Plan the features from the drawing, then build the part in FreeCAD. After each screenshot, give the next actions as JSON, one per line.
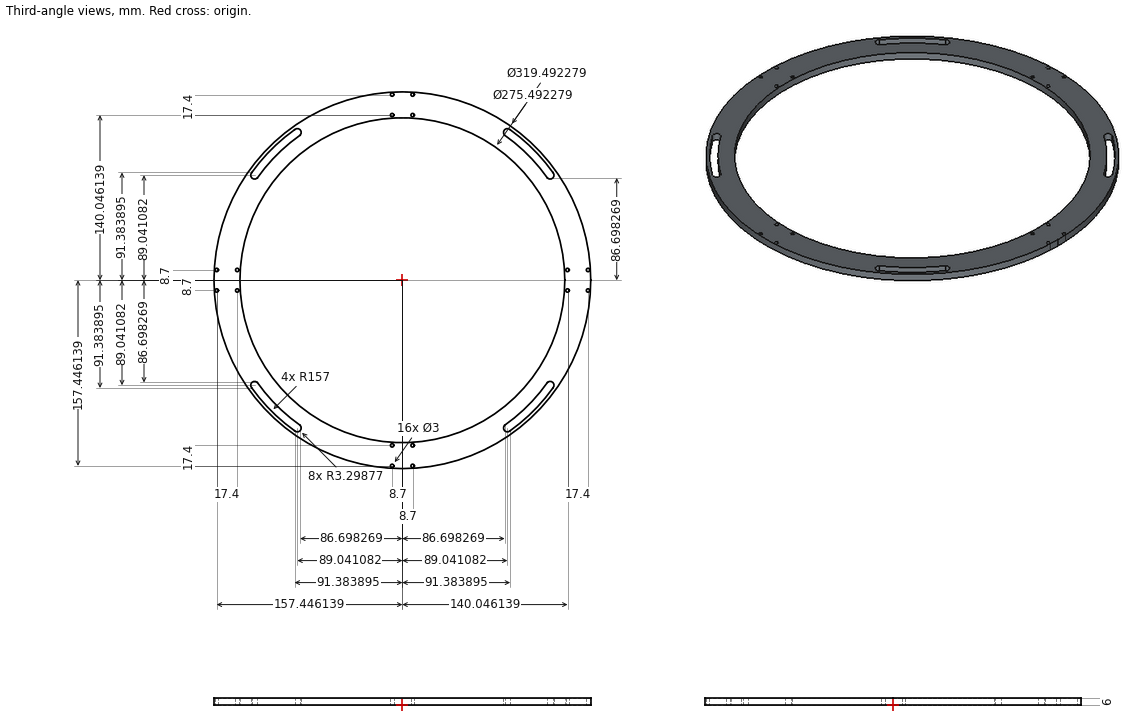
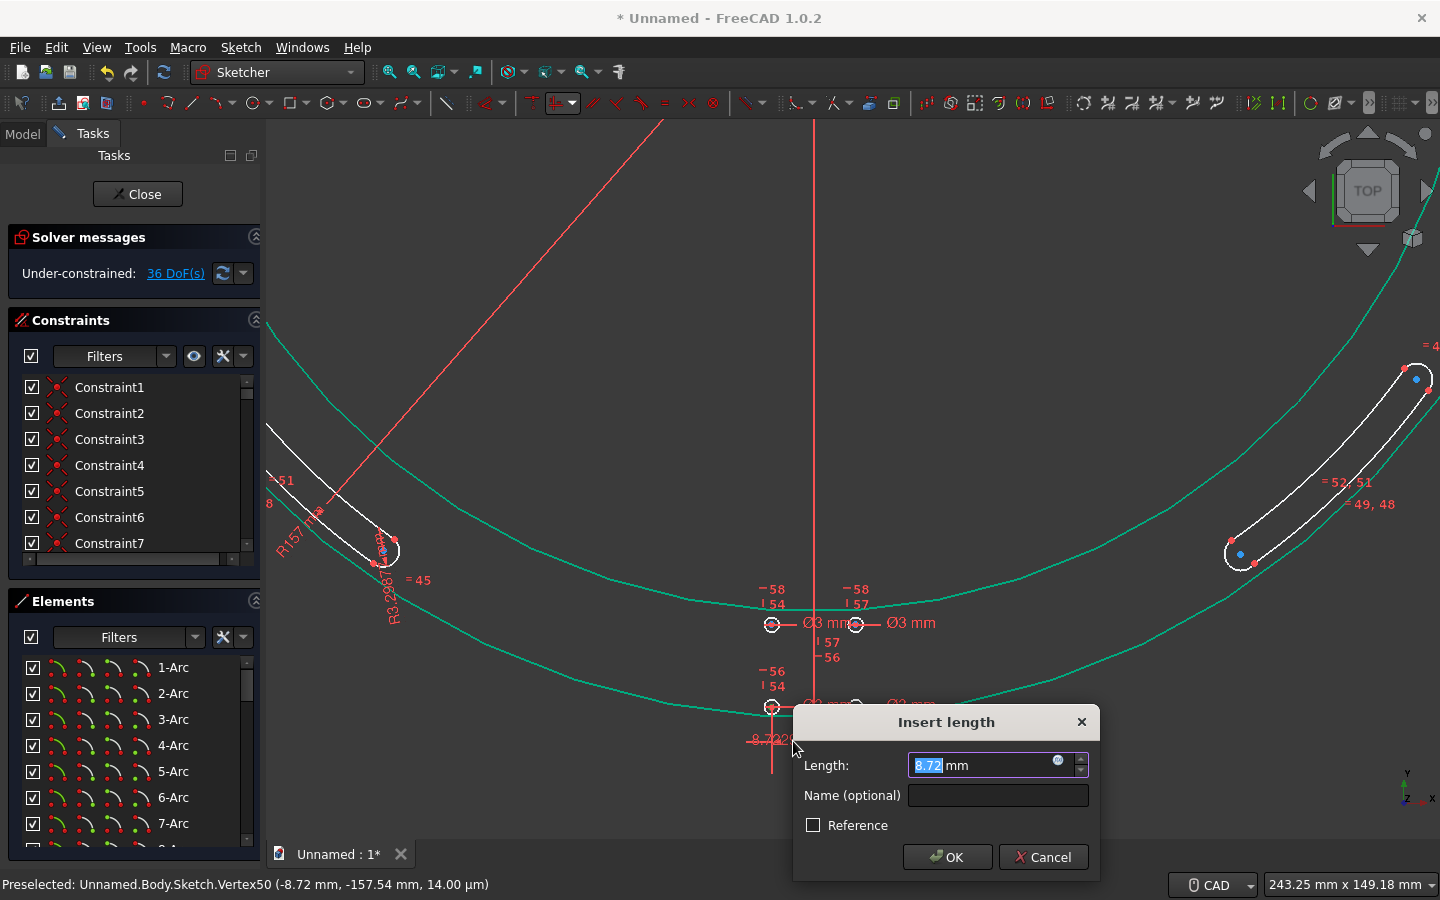
{"action": "type", "text": "8.7"}
{"action": "key", "text": "Return"}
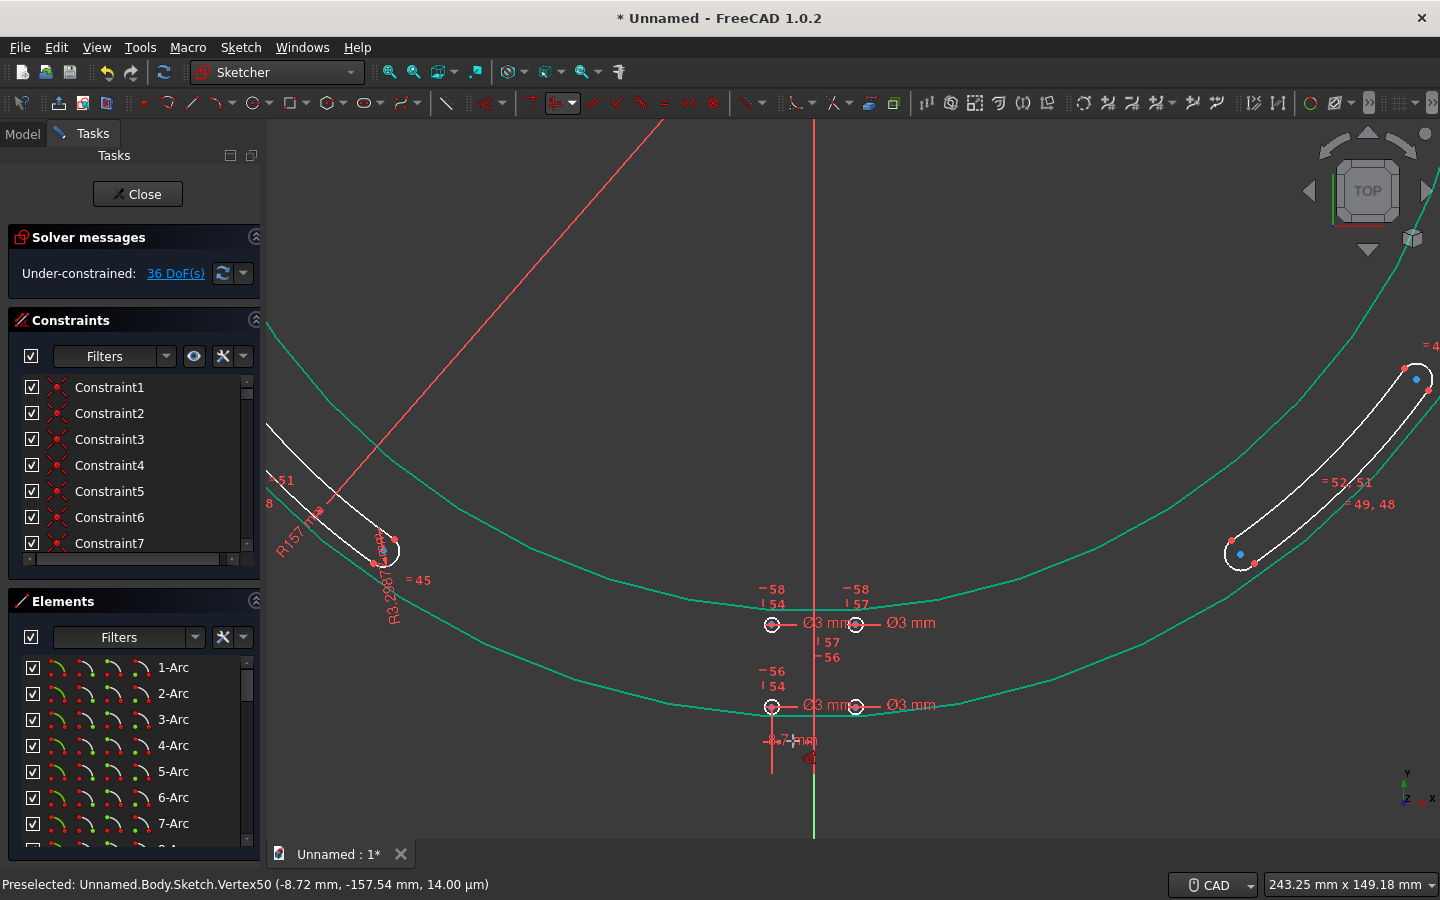
{"action": "scroll", "coordinate": [772, 708], "scroll_direction": "down", "scroll_amount": 6}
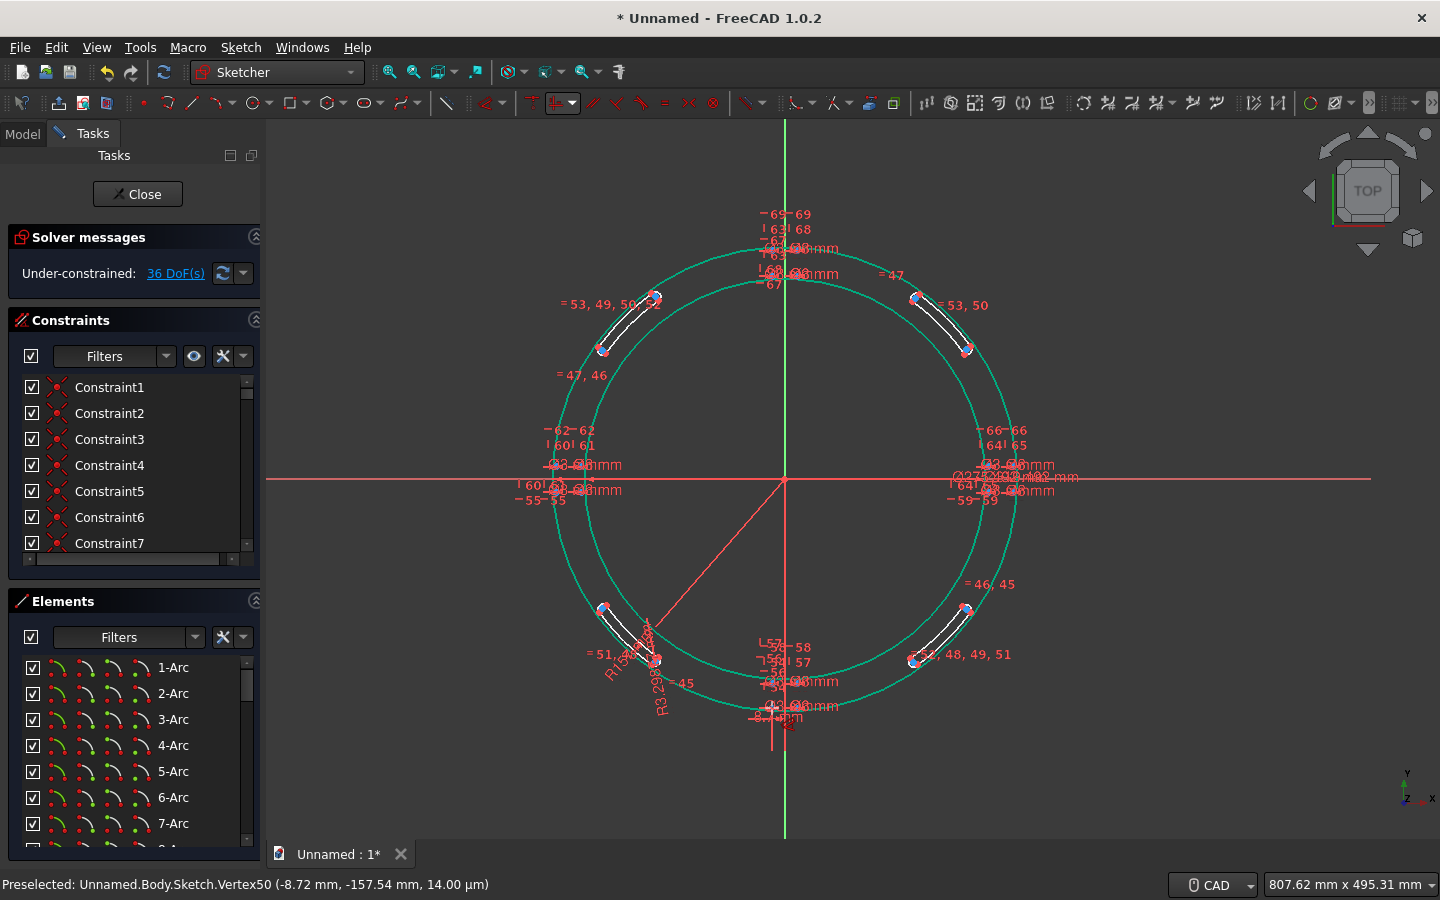
{"action": "scroll", "coordinate": [556, 492], "scroll_direction": "up", "scroll_amount": 6}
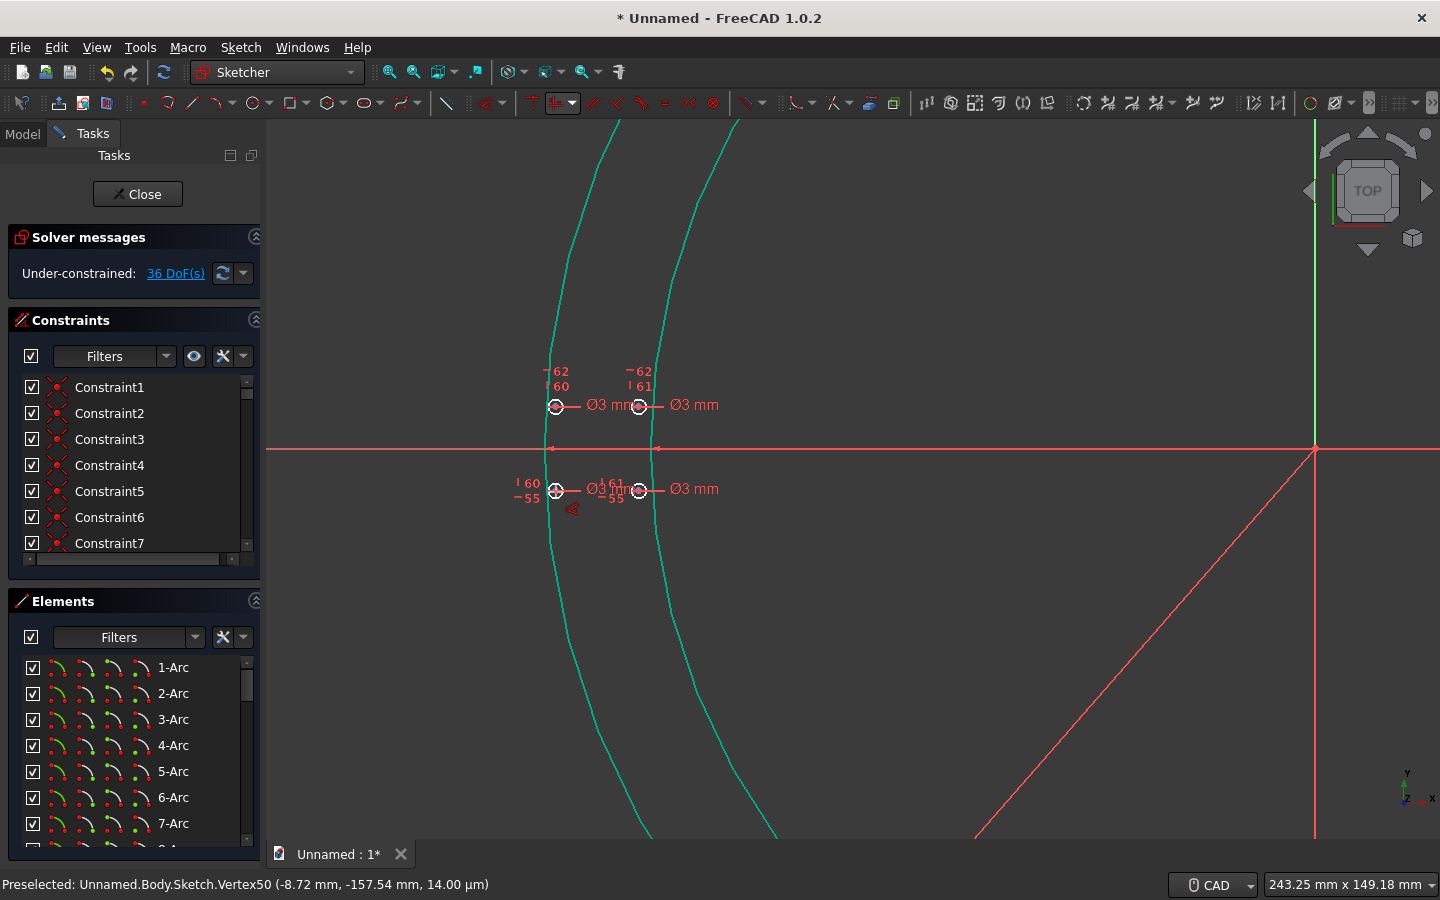
{"action": "left_click", "coordinate": [556, 491]}
{"action": "left_click", "coordinate": [522, 470]}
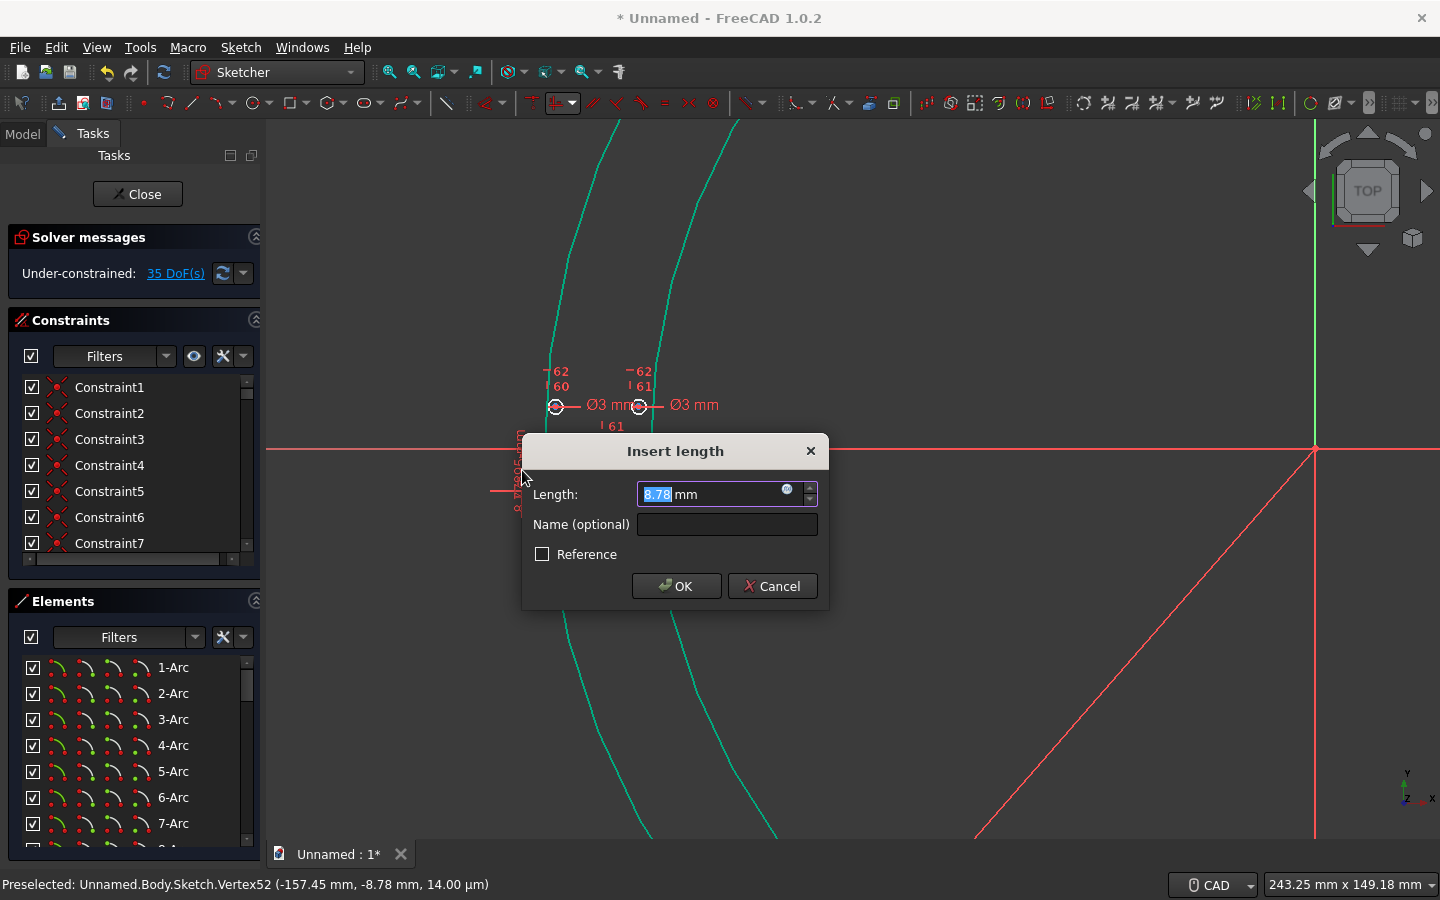
{"action": "type", "text": "8.7"}
{"action": "key", "text": "Return"}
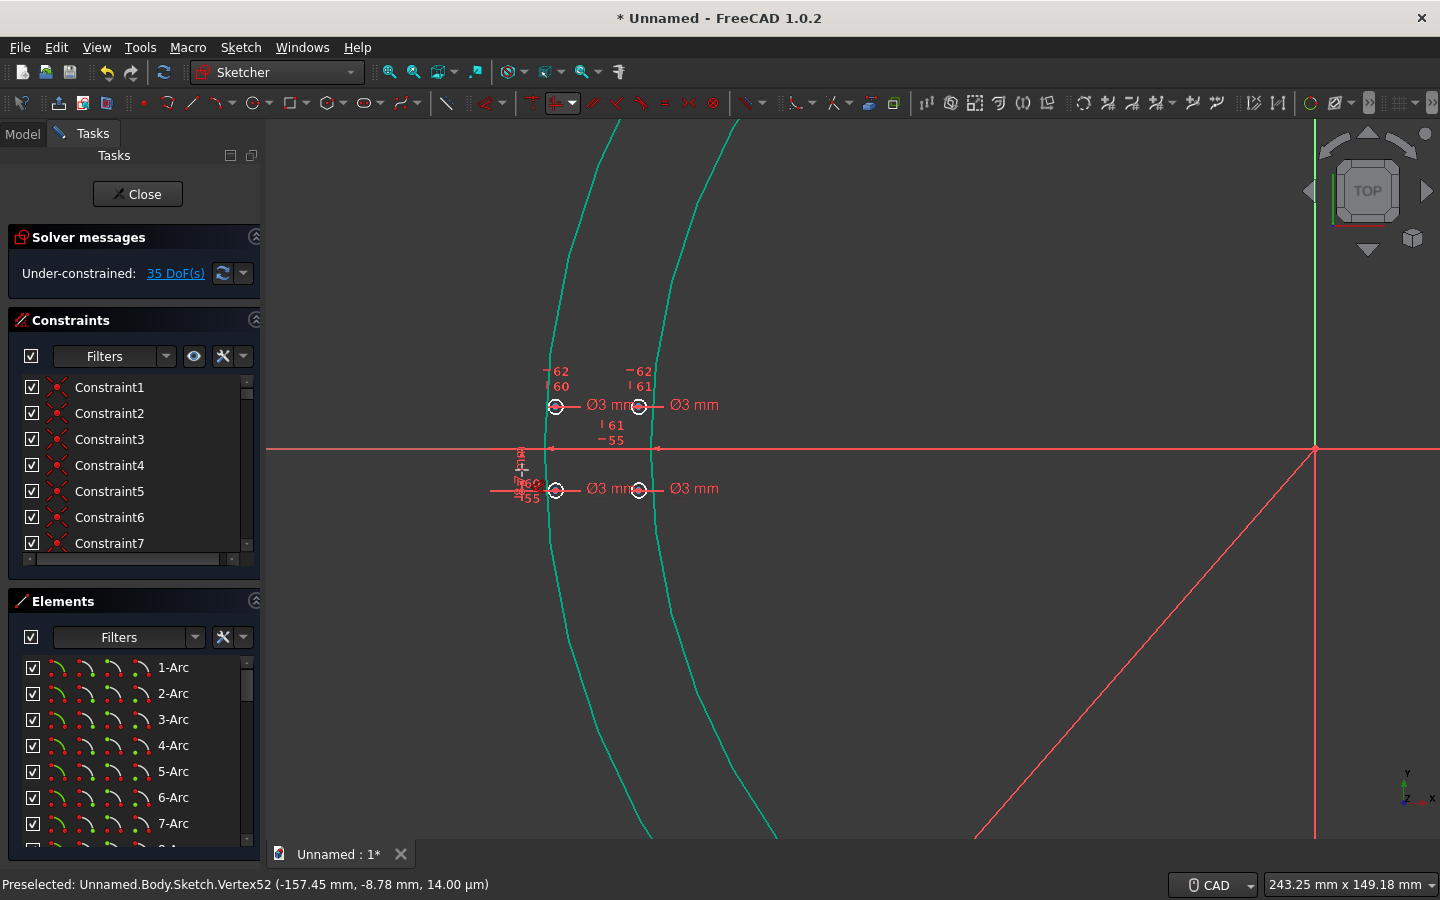
{"action": "scroll", "coordinate": [556, 492], "scroll_direction": "down", "scroll_amount": 6}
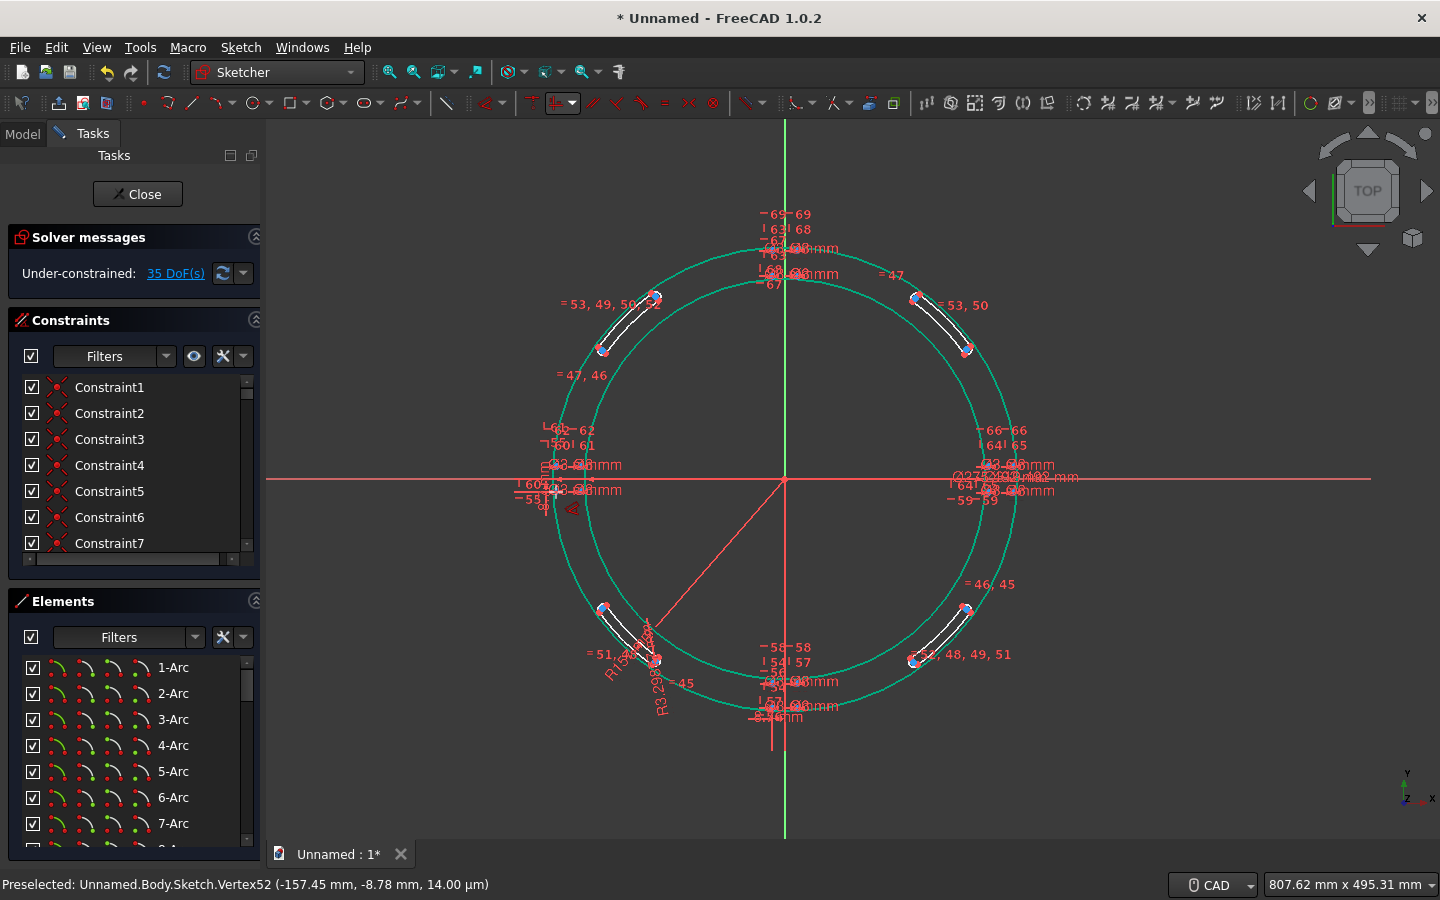
{"action": "scroll", "coordinate": [798, 708], "scroll_direction": "up", "scroll_amount": 6}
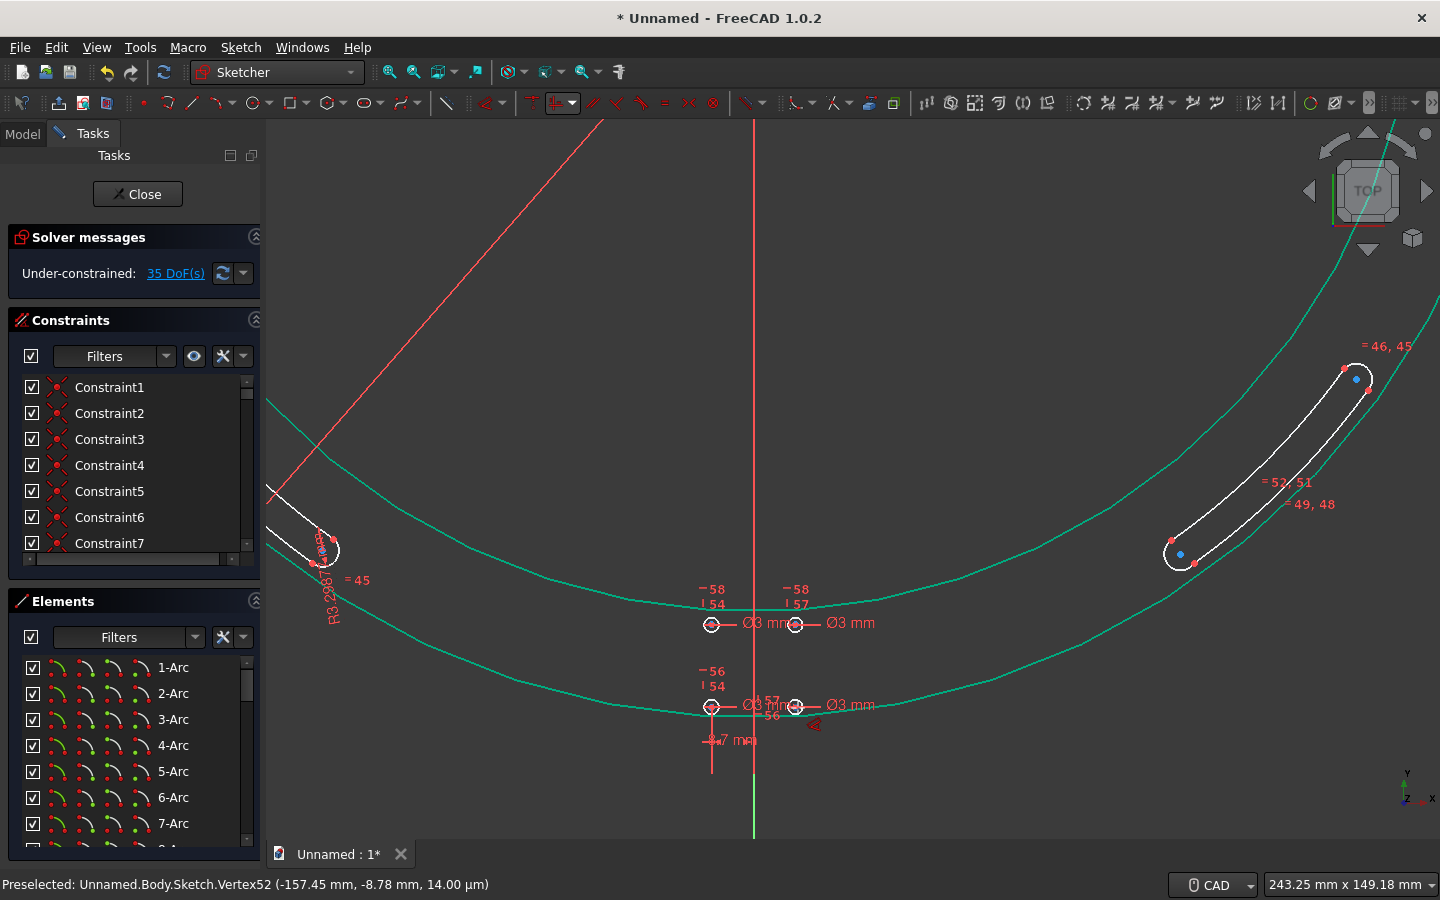
{"action": "left_click", "coordinate": [795, 707]}
{"action": "left_click", "coordinate": [774, 765]}